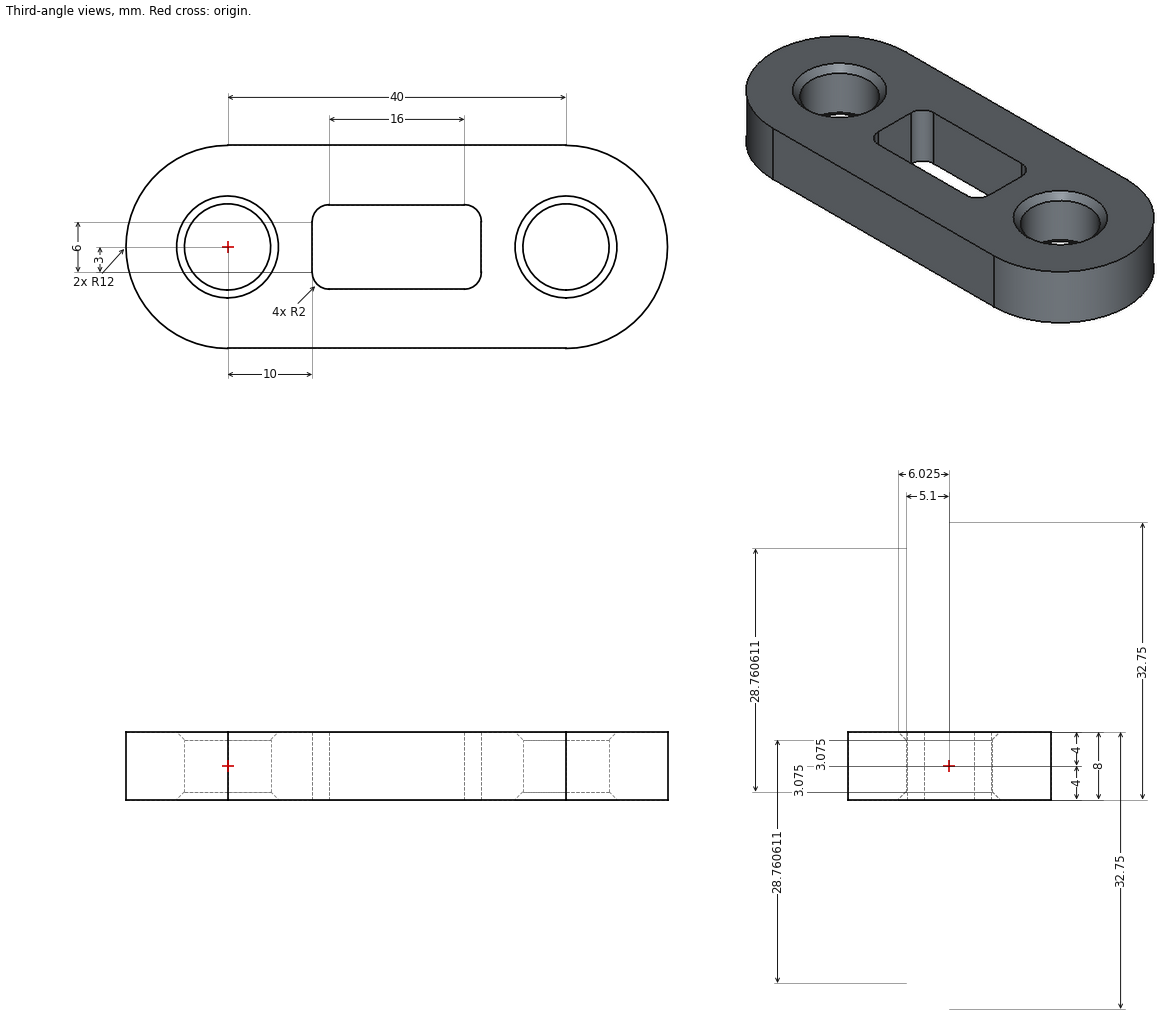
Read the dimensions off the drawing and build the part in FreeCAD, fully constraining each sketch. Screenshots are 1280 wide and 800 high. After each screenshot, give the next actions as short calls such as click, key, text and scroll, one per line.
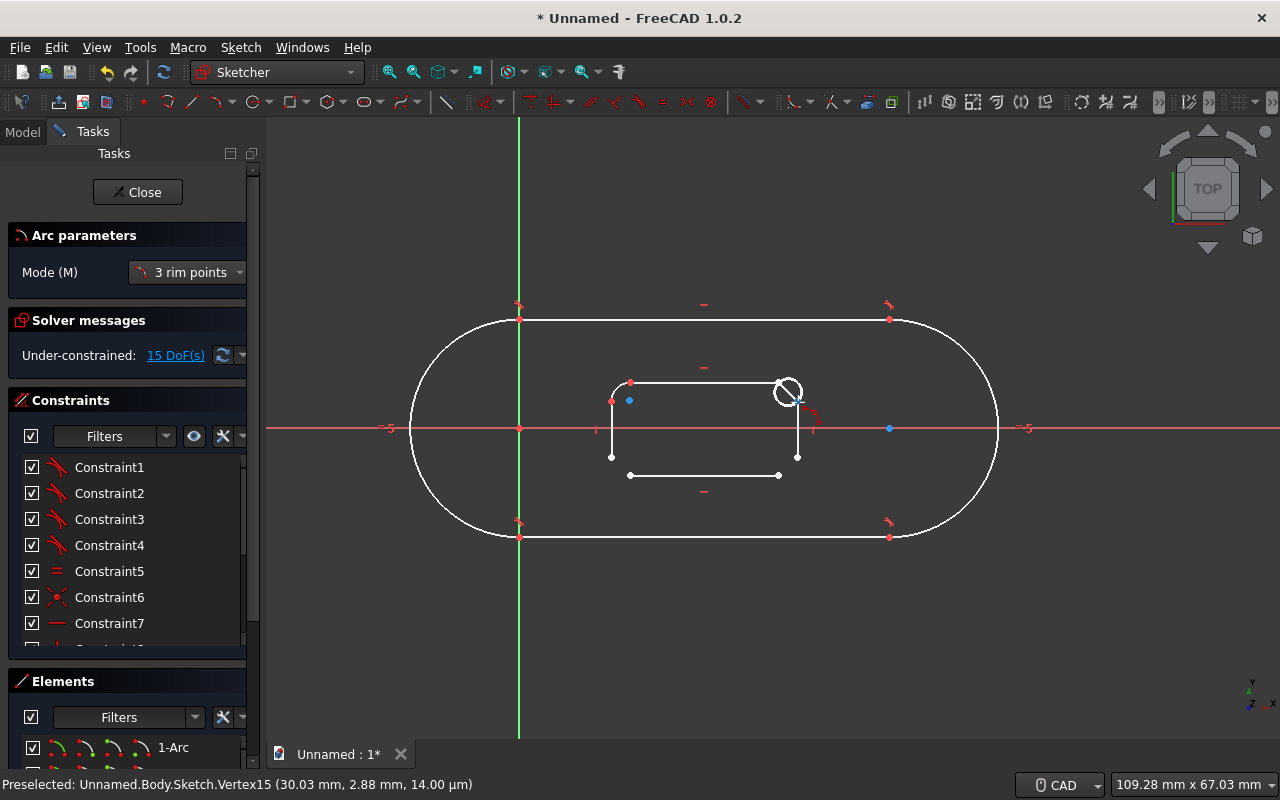
scroll(792, 387, up, 6)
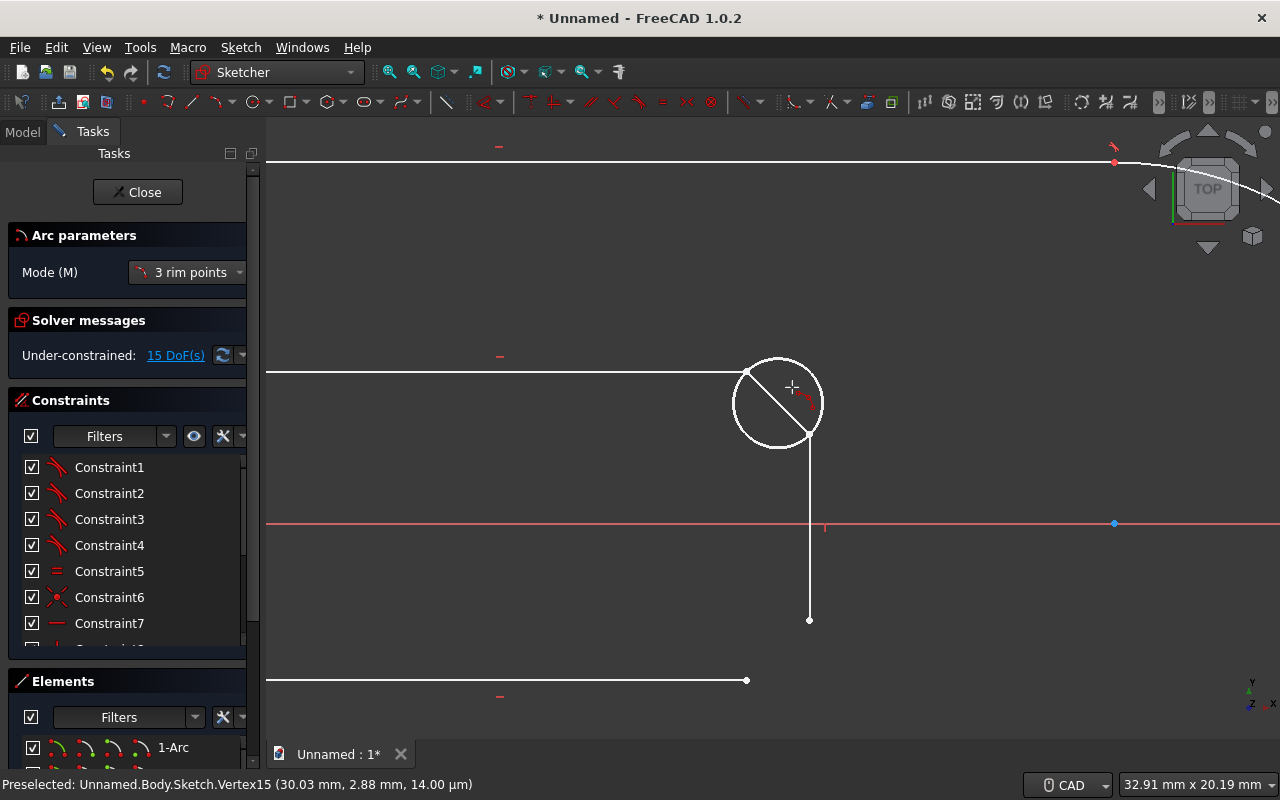
click(791, 388)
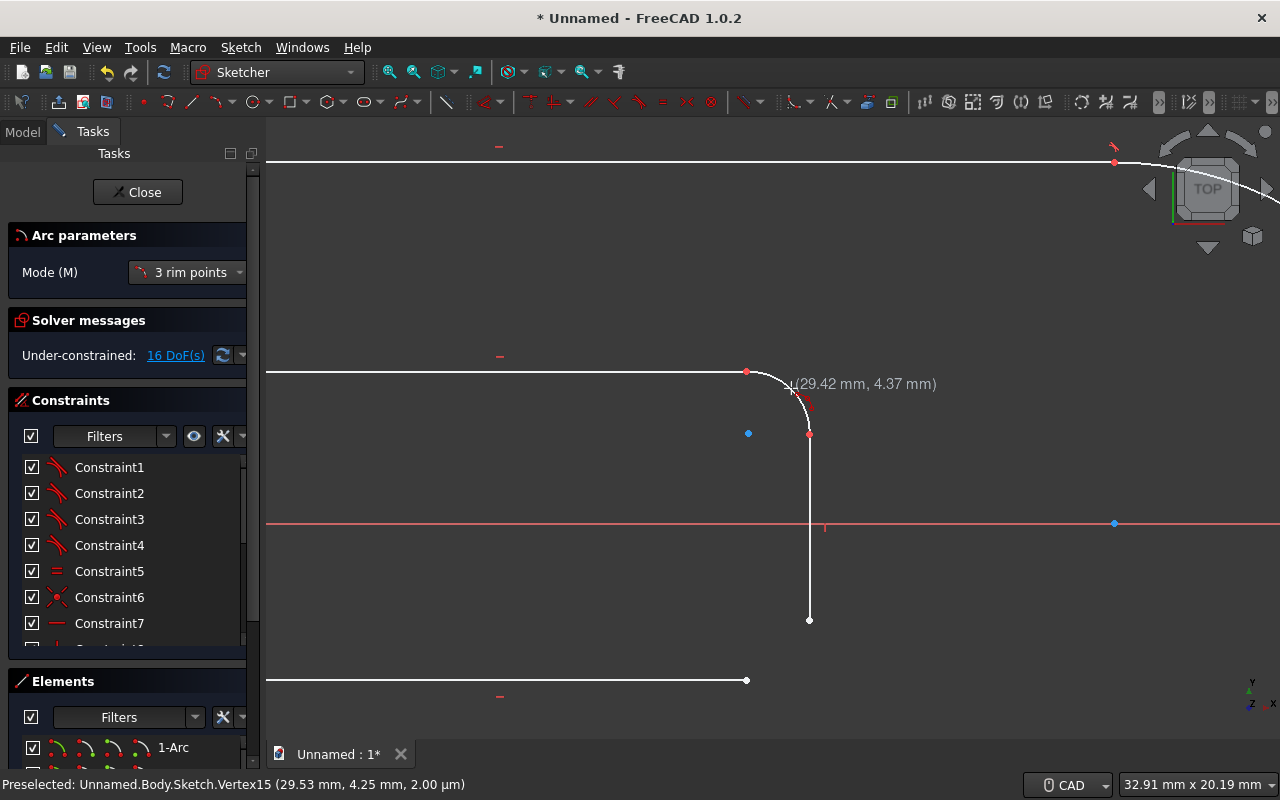
click(810, 621)
click(747, 680)
click(791, 660)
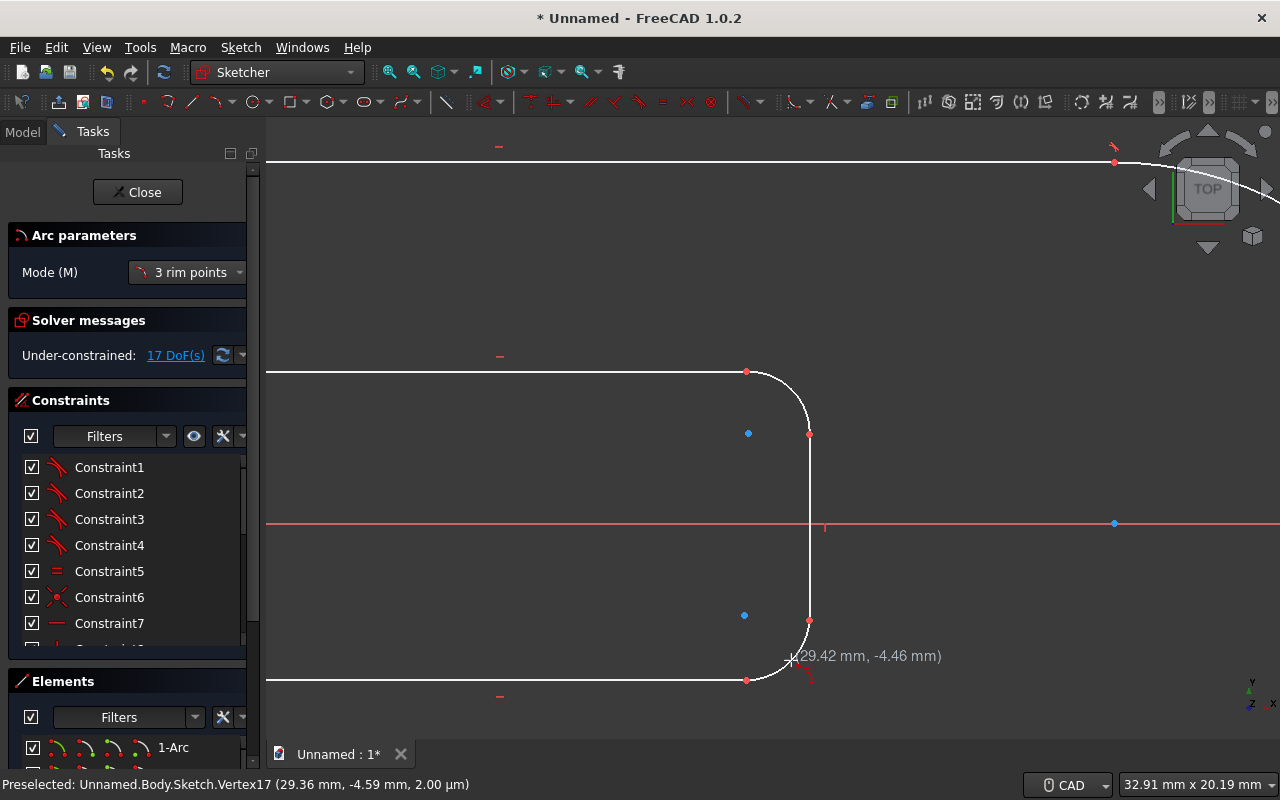
scroll(792, 387, down, 6)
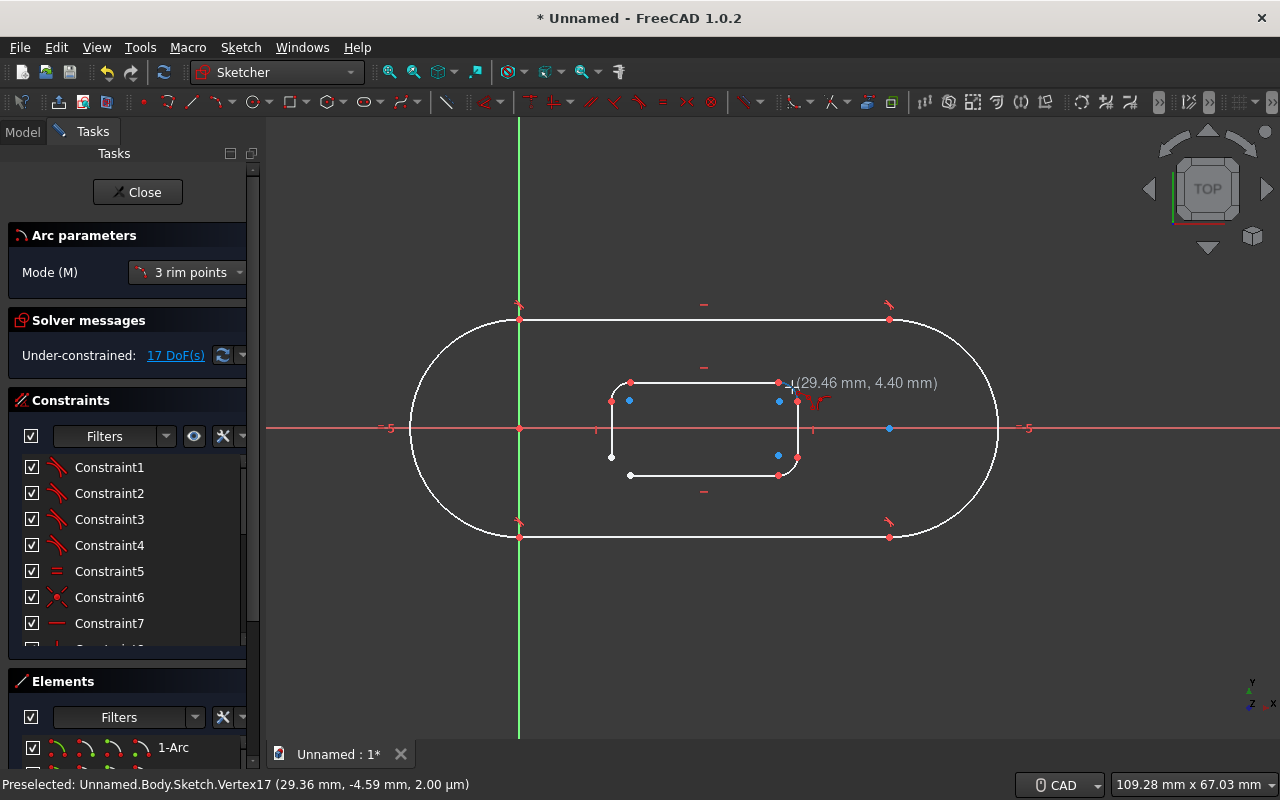
click(631, 476)
click(612, 458)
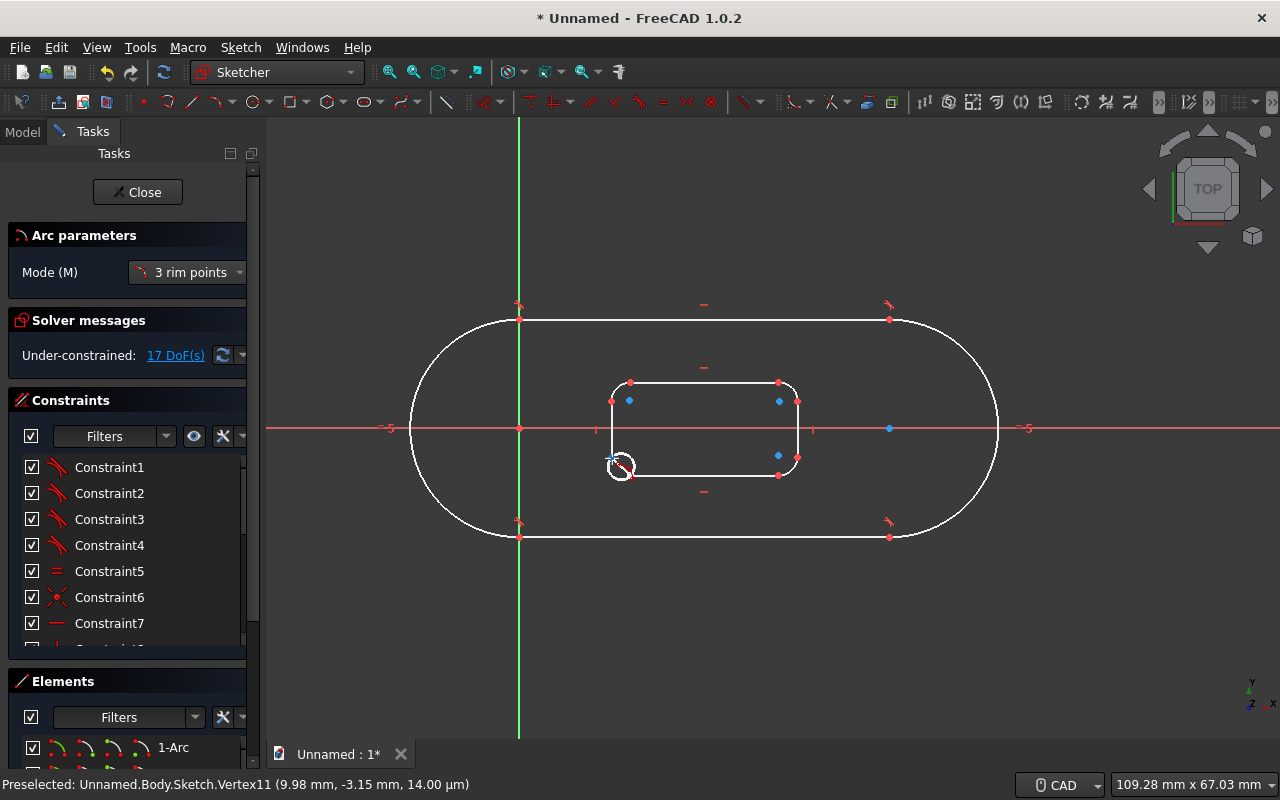
scroll(617, 469, up, 6)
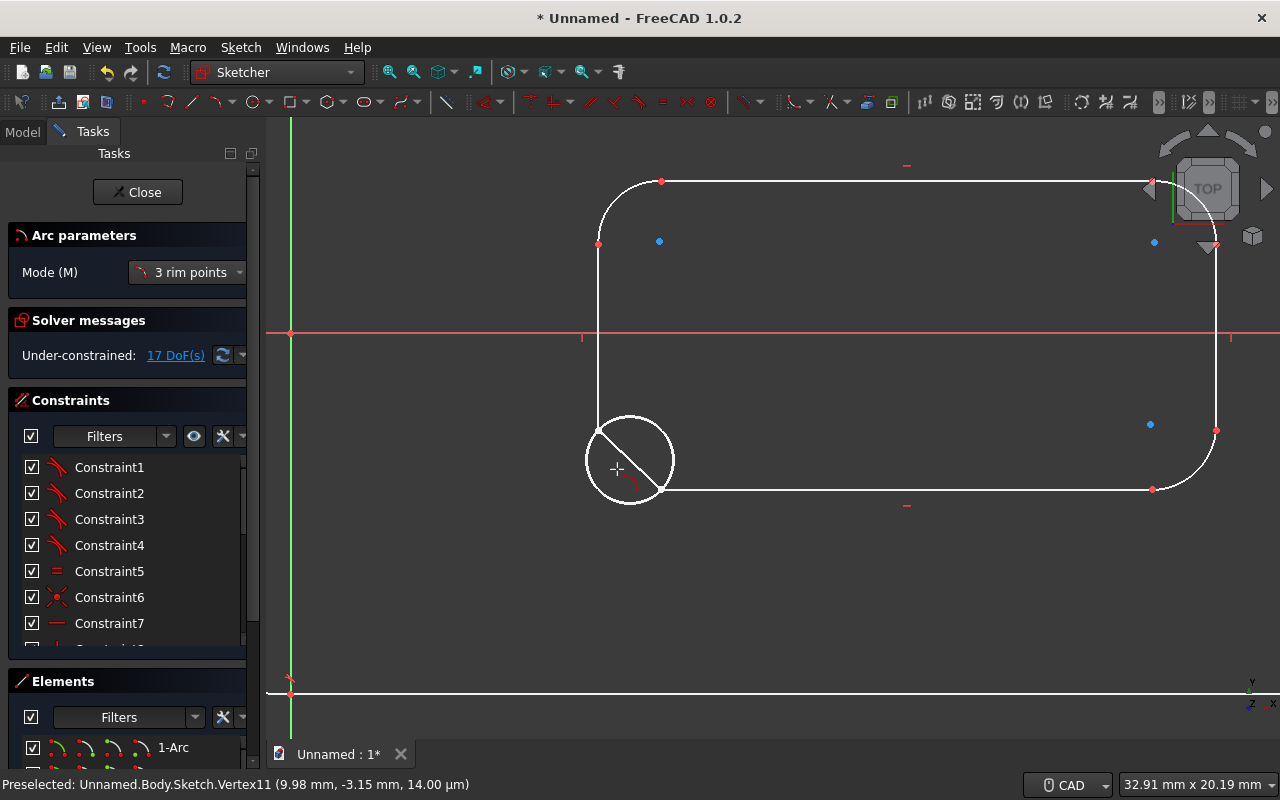
click(617, 469)
key(Escape)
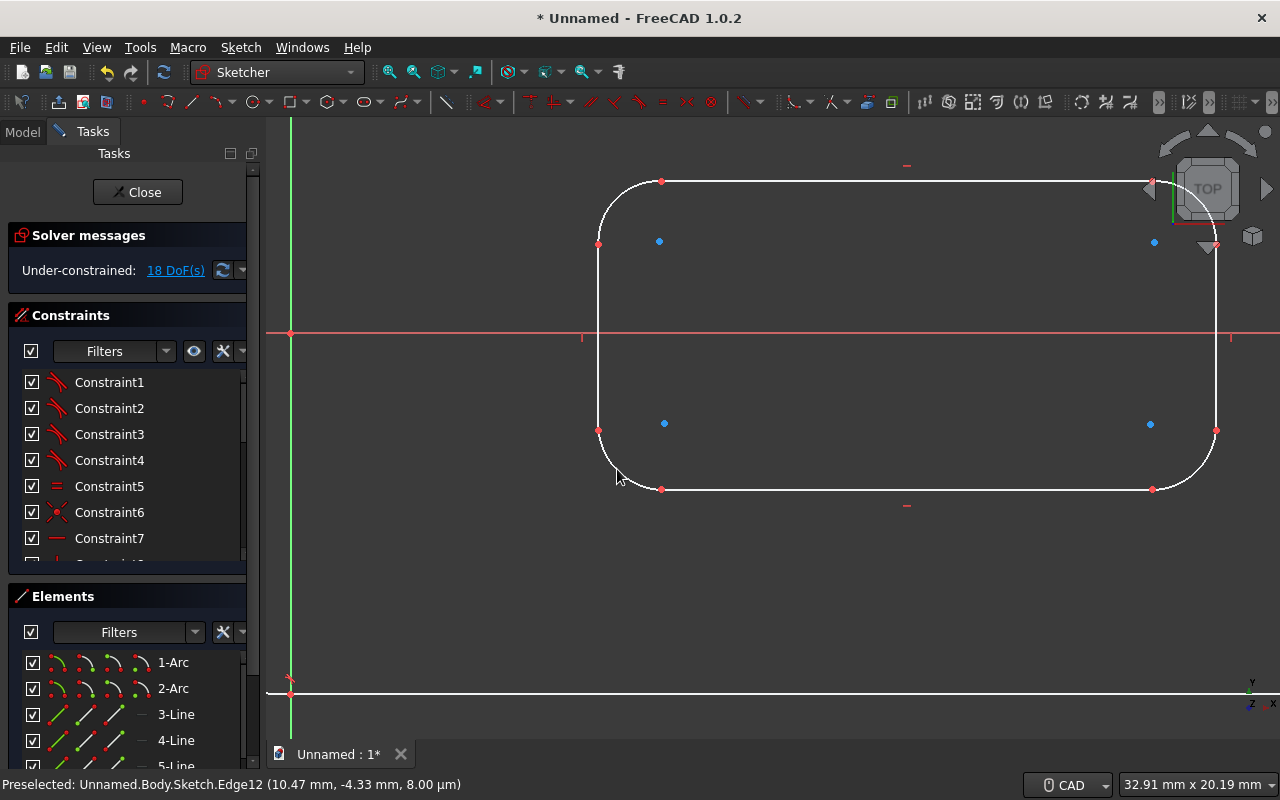
click(598, 374)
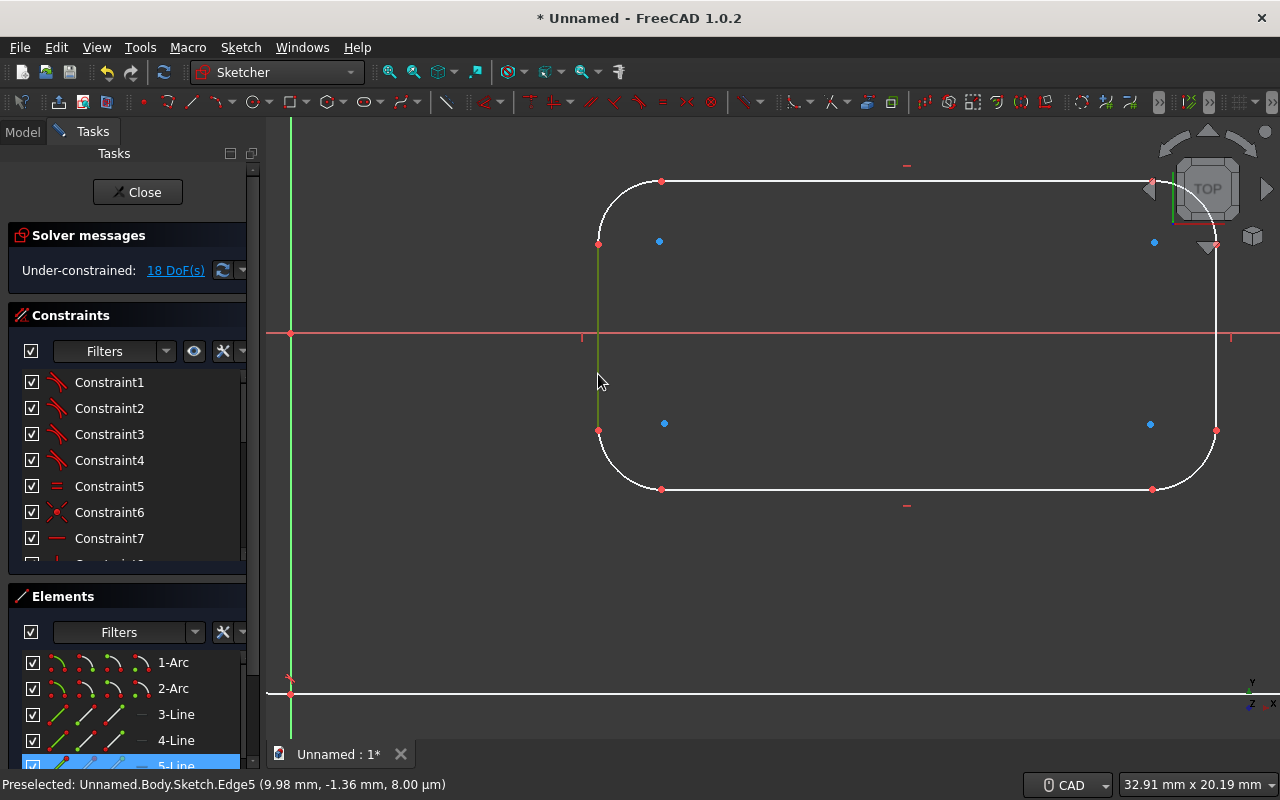
click(632, 187)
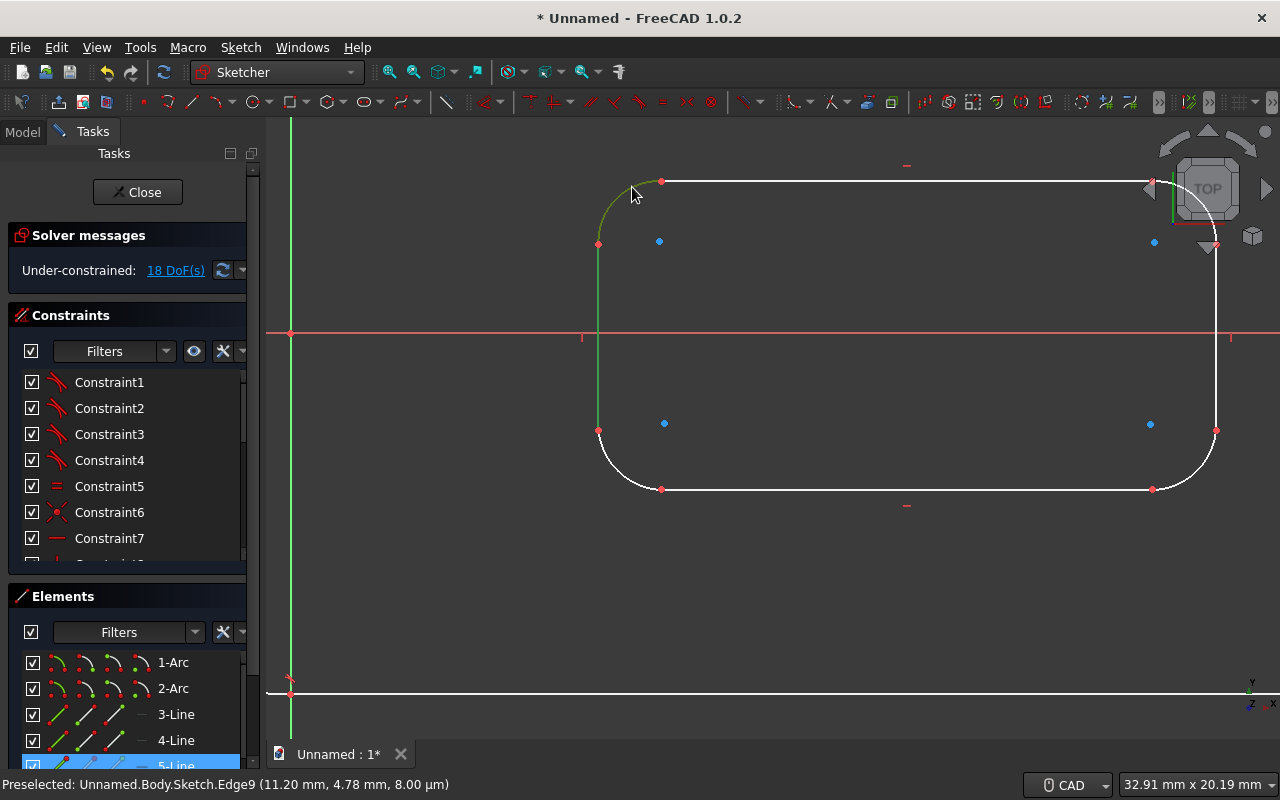
key(t)